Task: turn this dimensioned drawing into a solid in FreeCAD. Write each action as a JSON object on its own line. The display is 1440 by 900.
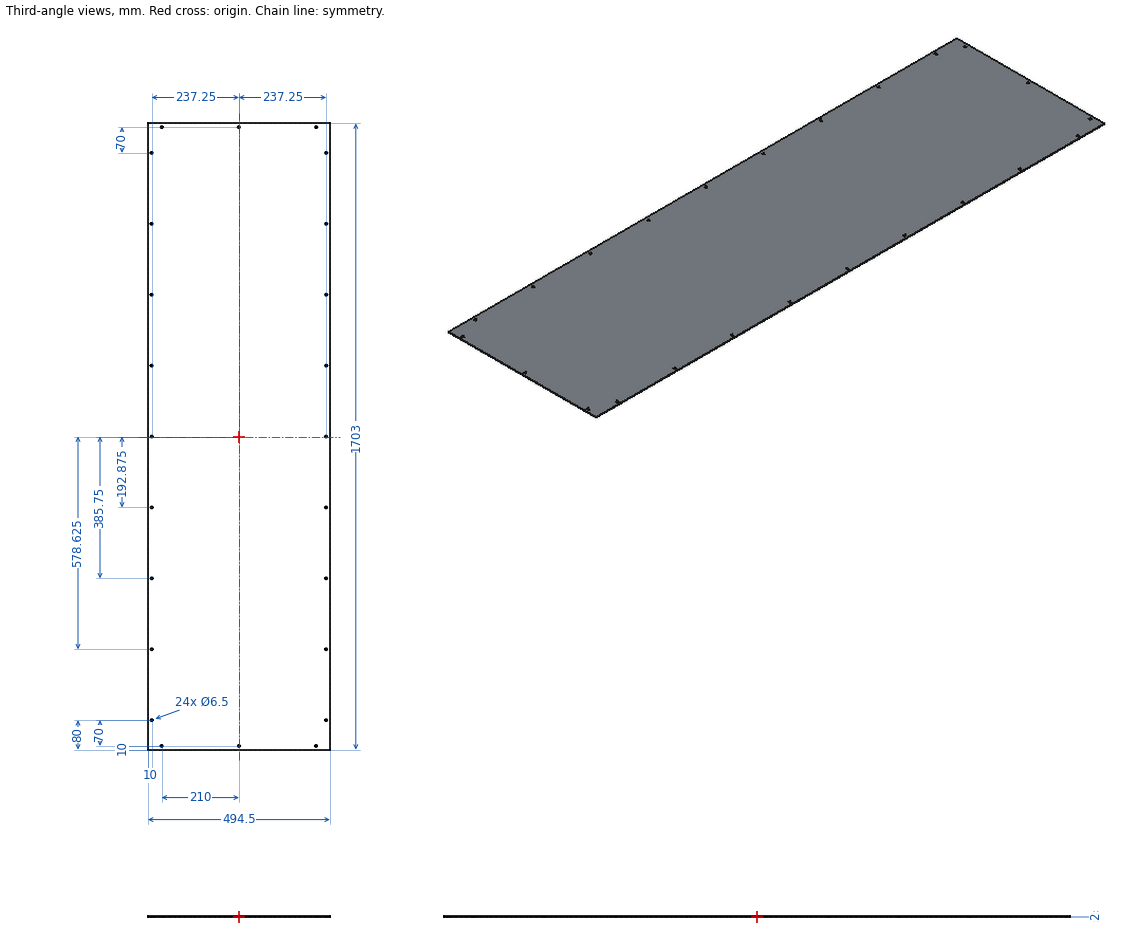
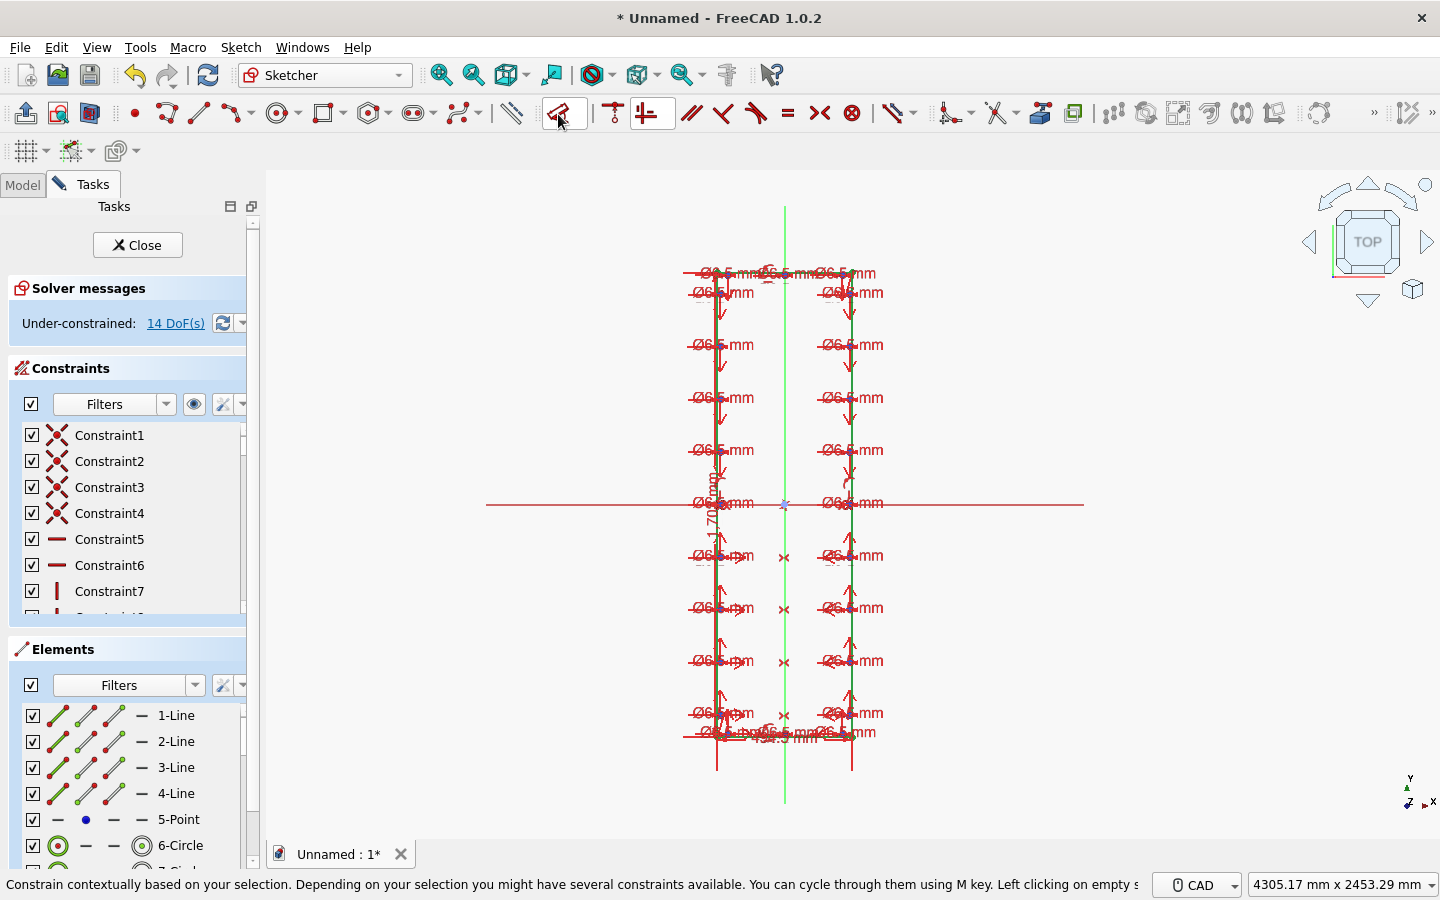
{"action": "left_click", "coordinate": [728, 734]}
{"action": "left_click", "coordinate": [756, 768]}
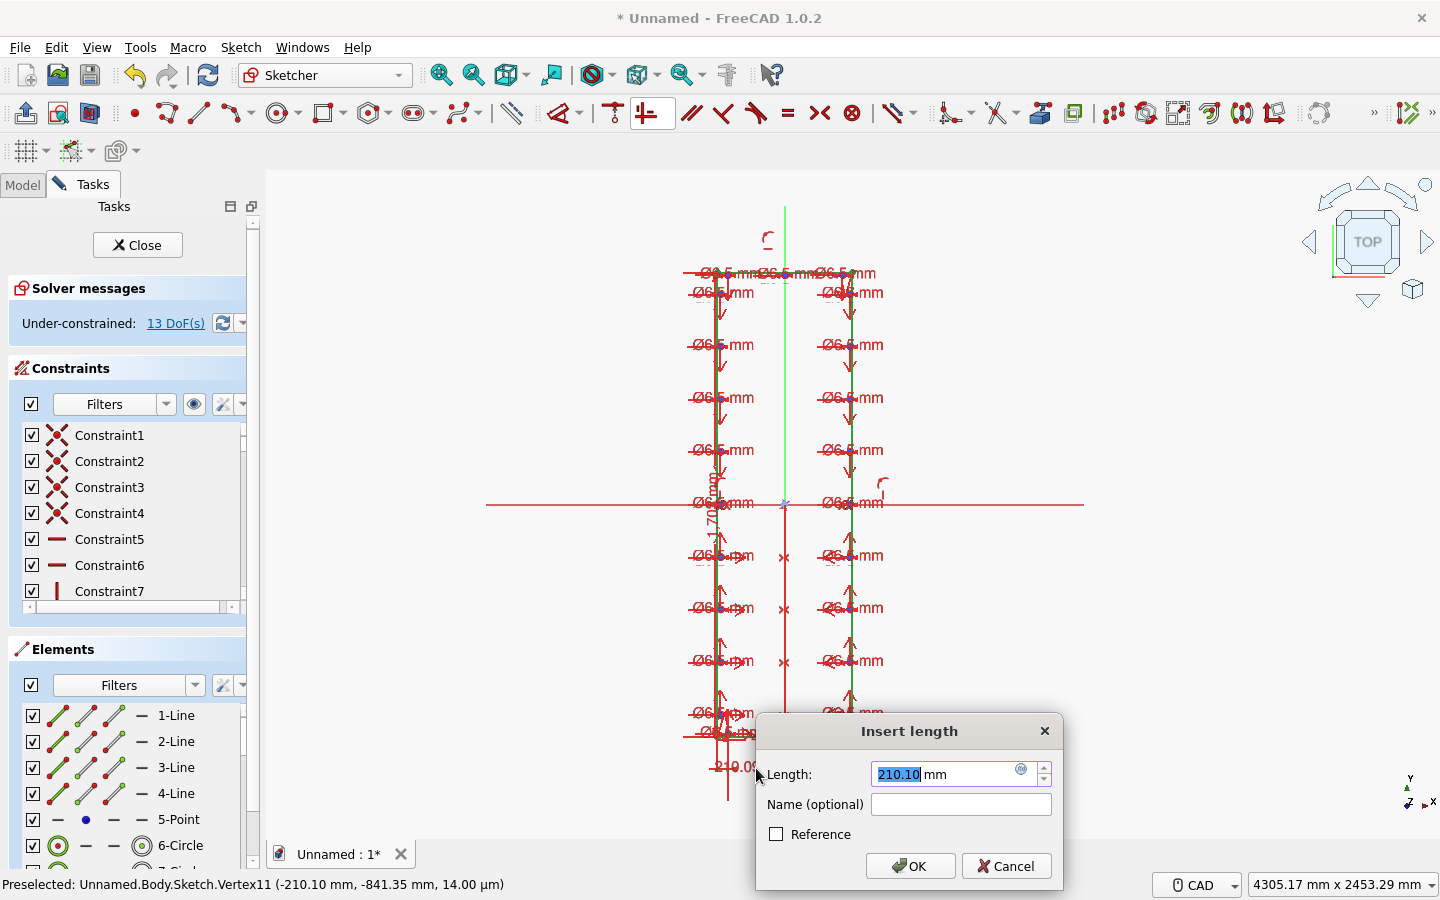
{"action": "type", "text": "210"}
{"action": "key", "text": "Return"}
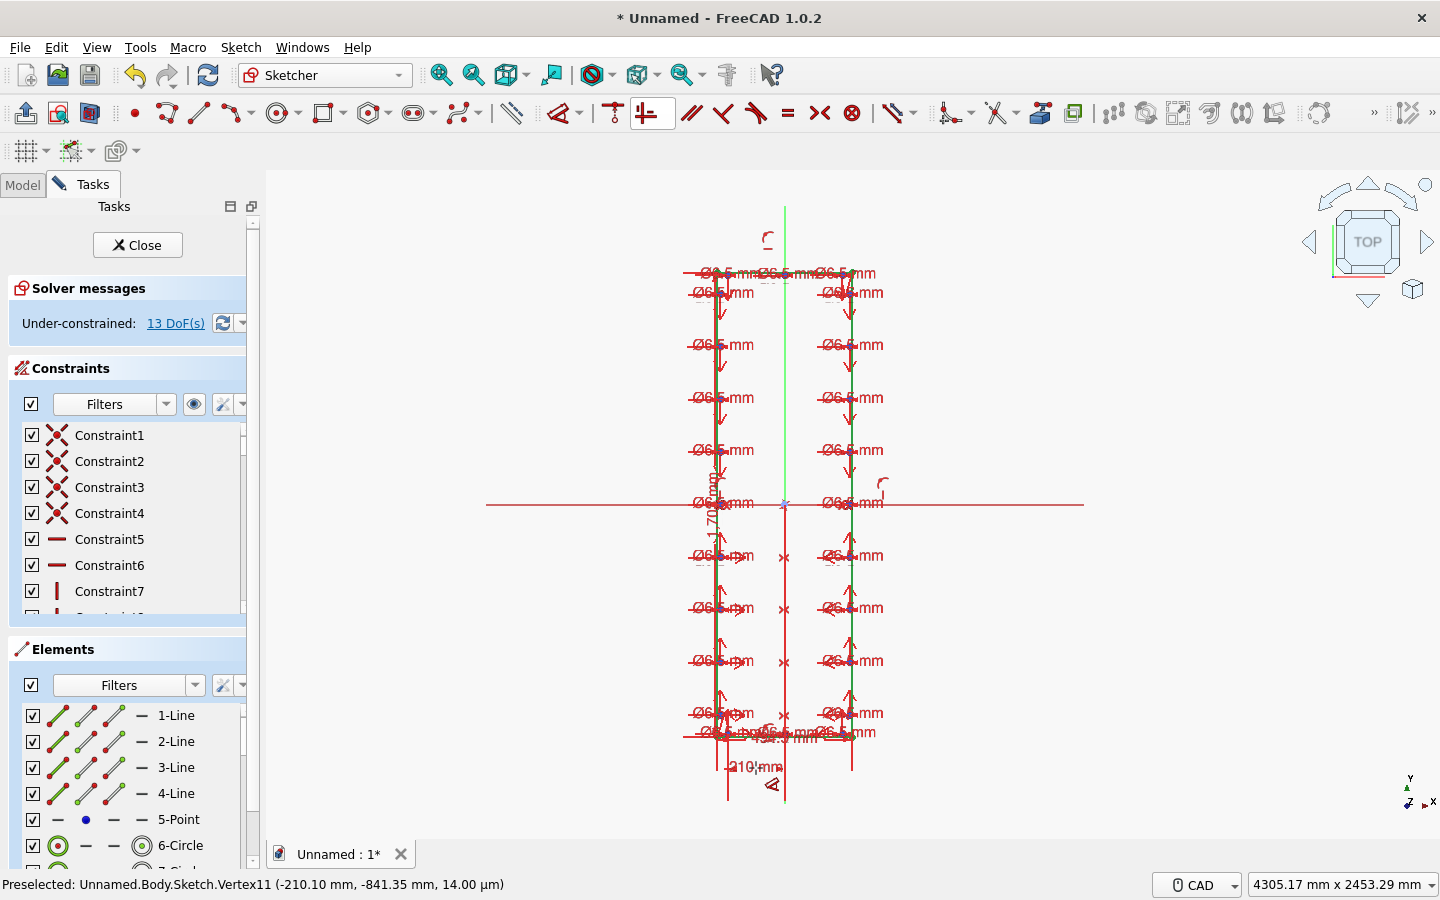
{"action": "scroll", "coordinate": [717, 737], "scroll_direction": "up", "scroll_amount": 14}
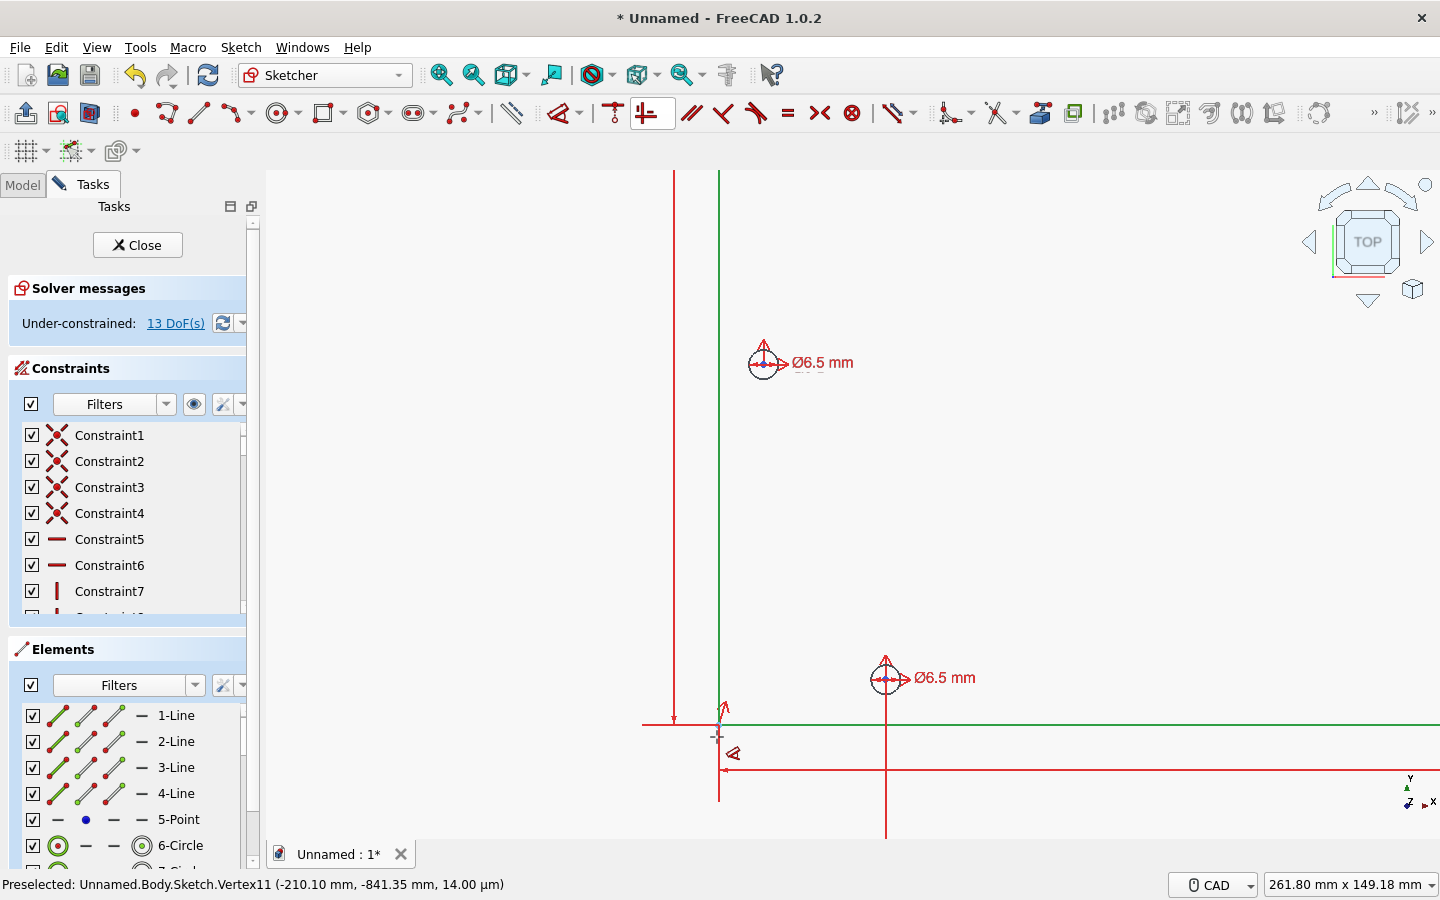
{"action": "left_click", "coordinate": [719, 725]}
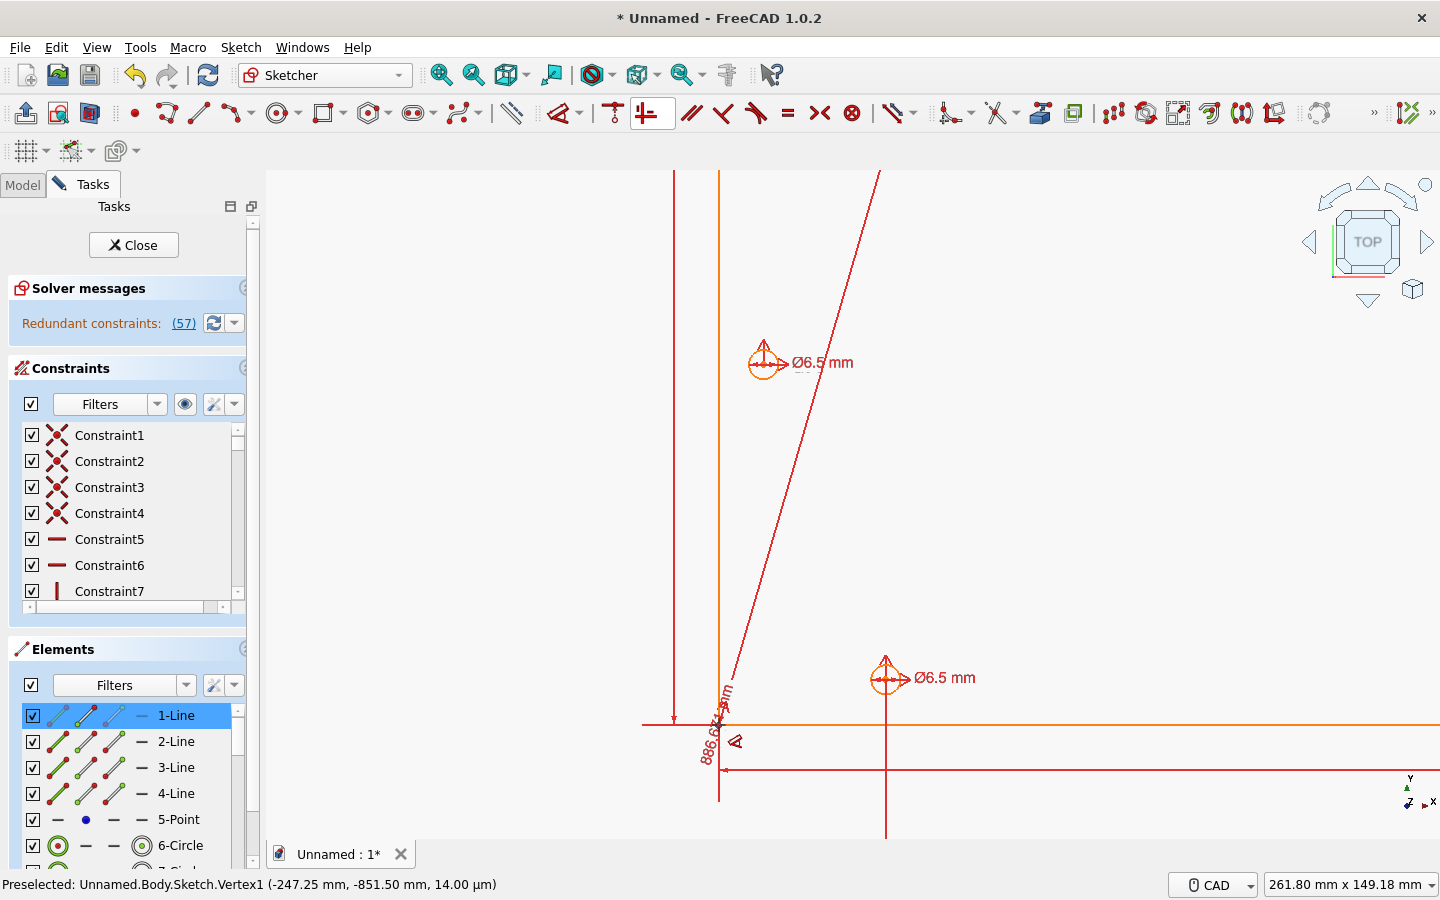
{"action": "left_click", "coordinate": [764, 365]}
{"action": "left_click", "coordinate": [741, 759]}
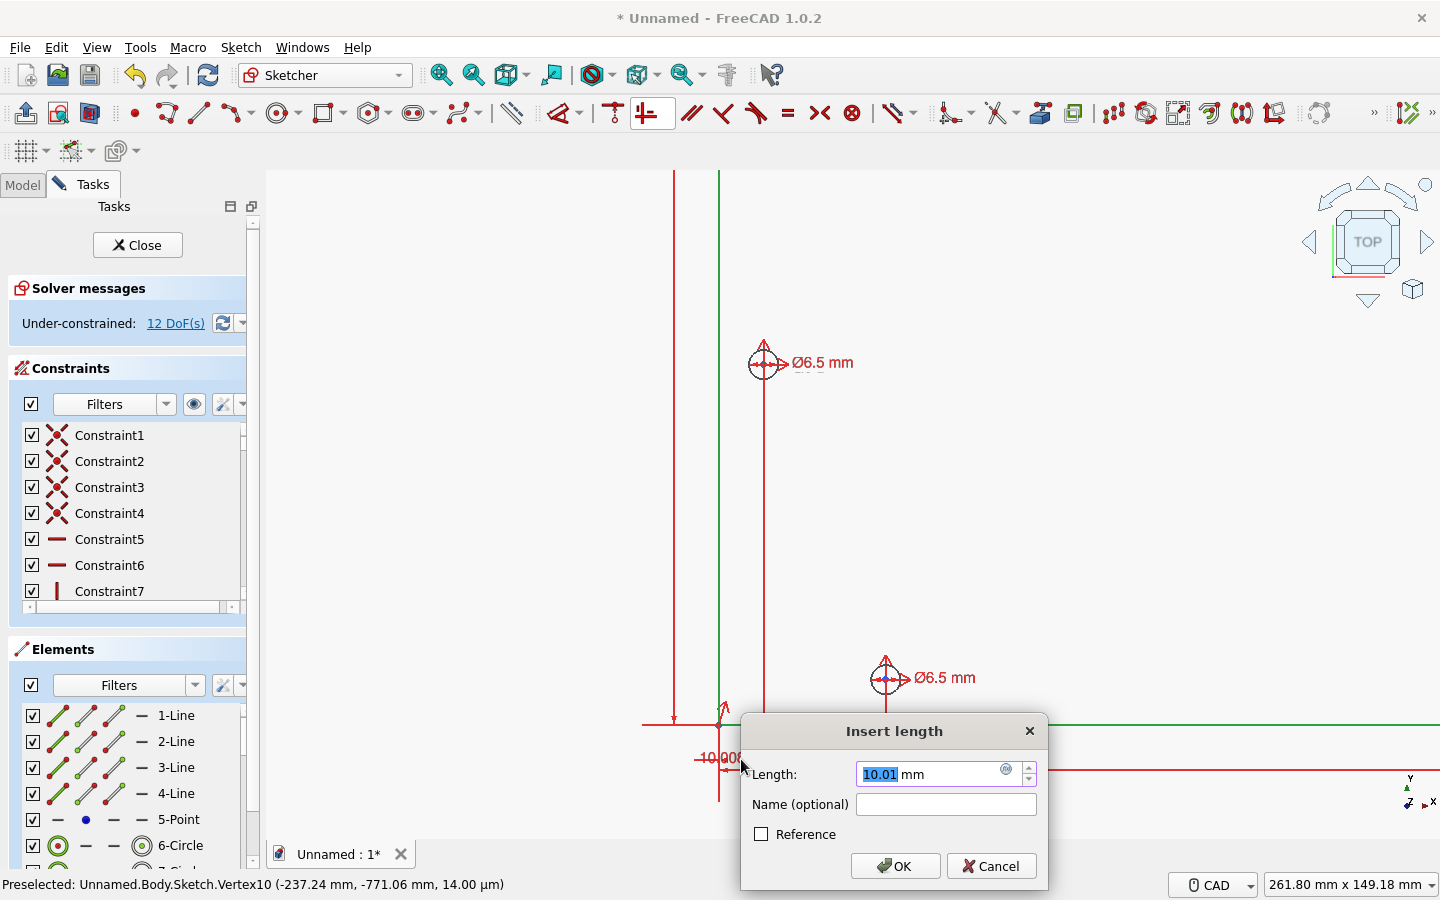
{"action": "type", "text": "10"}
{"action": "key", "text": "Return"}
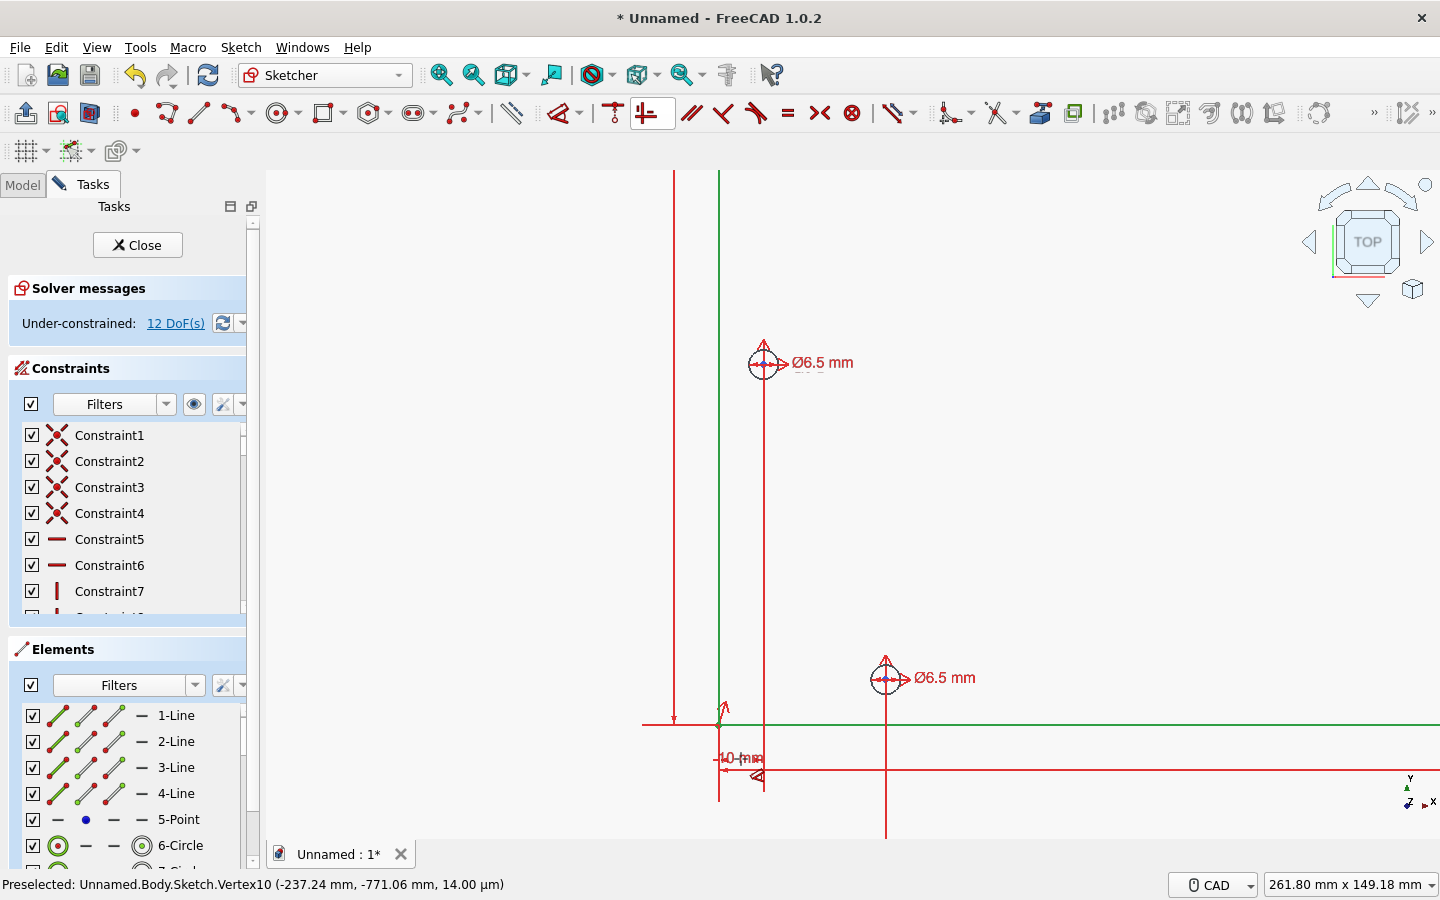
{"action": "scroll", "coordinate": [717, 737], "scroll_direction": "down", "scroll_amount": 14}